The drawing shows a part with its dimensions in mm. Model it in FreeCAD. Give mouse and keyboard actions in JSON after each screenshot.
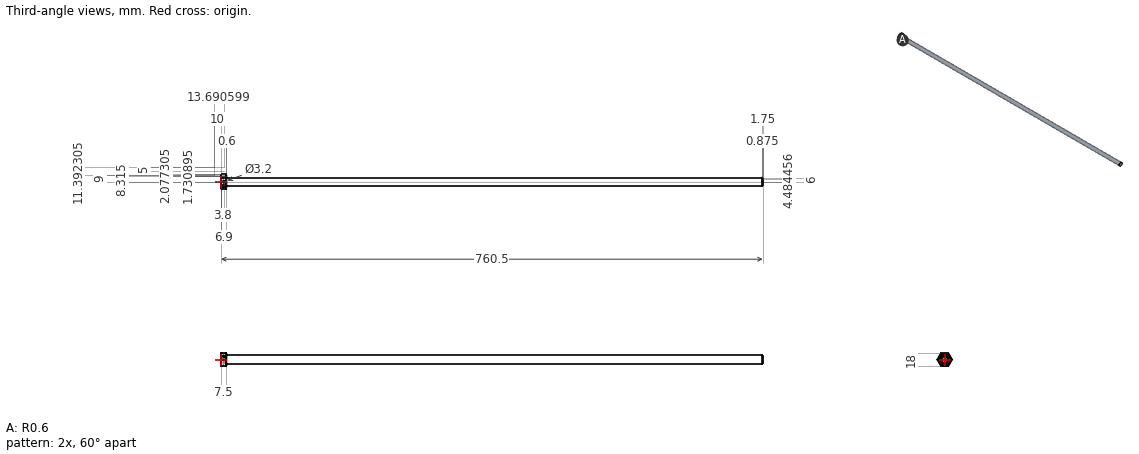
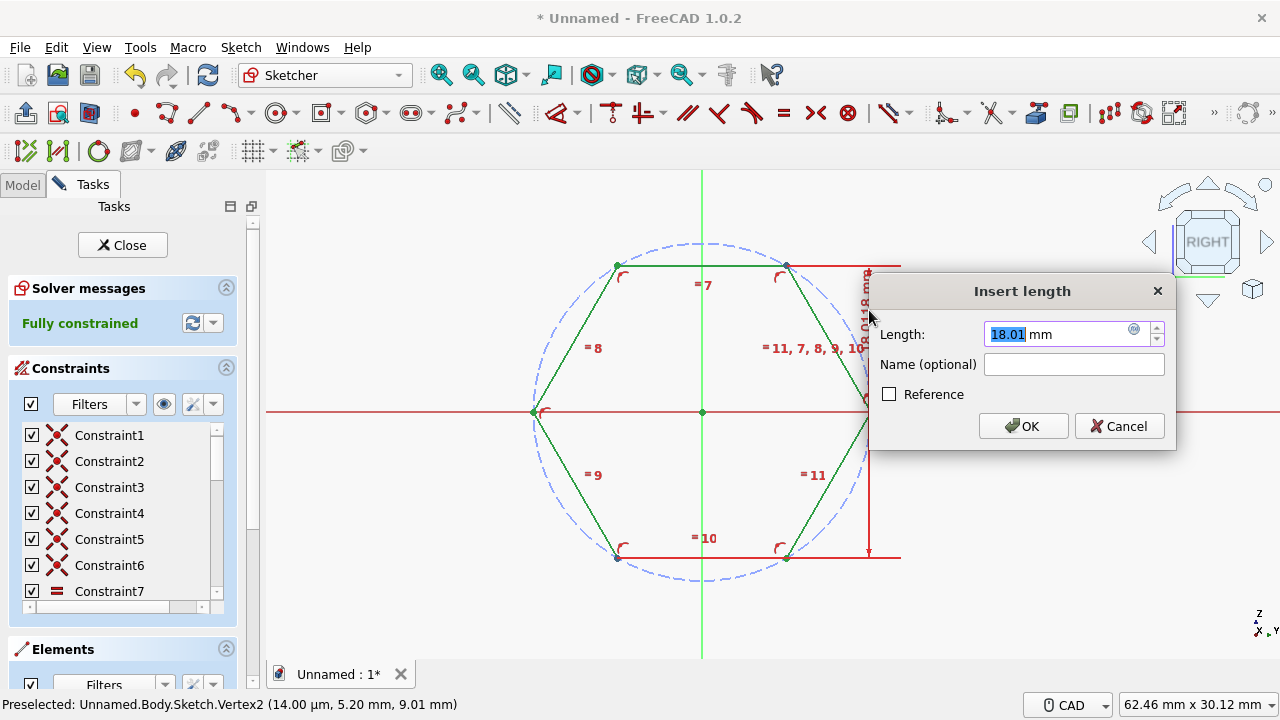
{"action": "type", "text": "18"}
{"action": "key", "text": "Return"}
{"action": "key", "text": "Escape"}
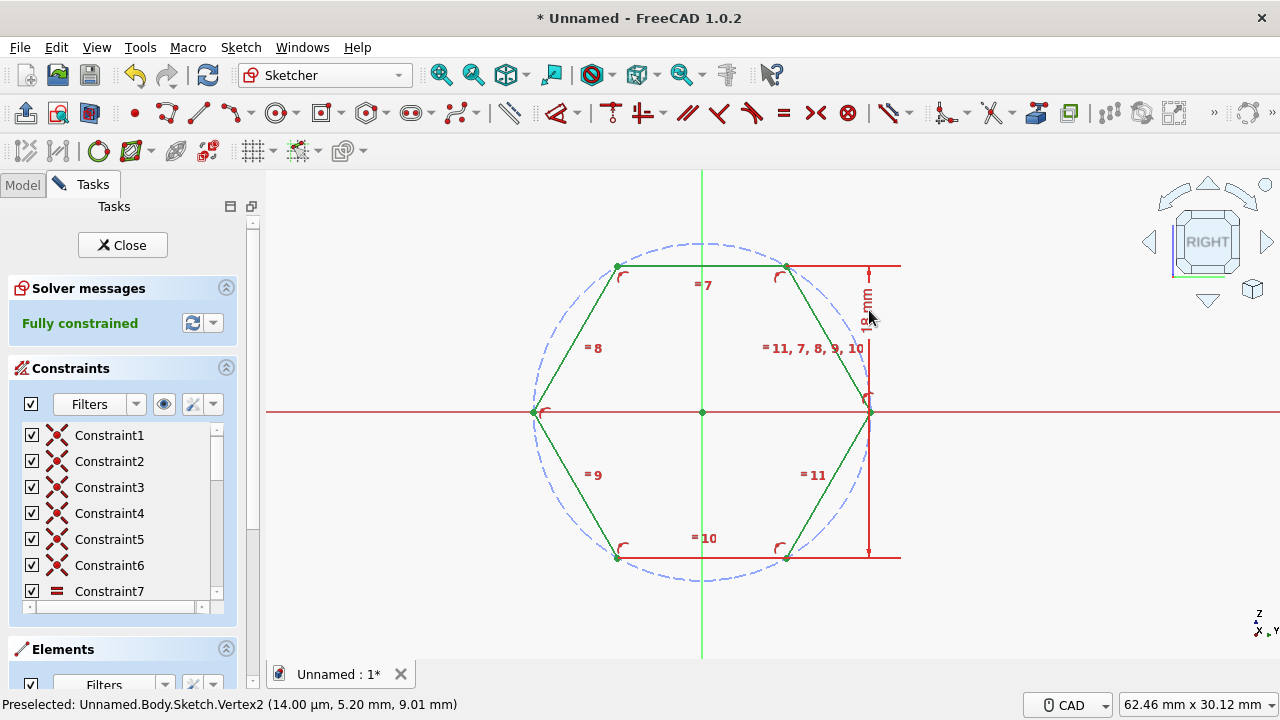
{"action": "left_click", "coordinate": [123, 245]}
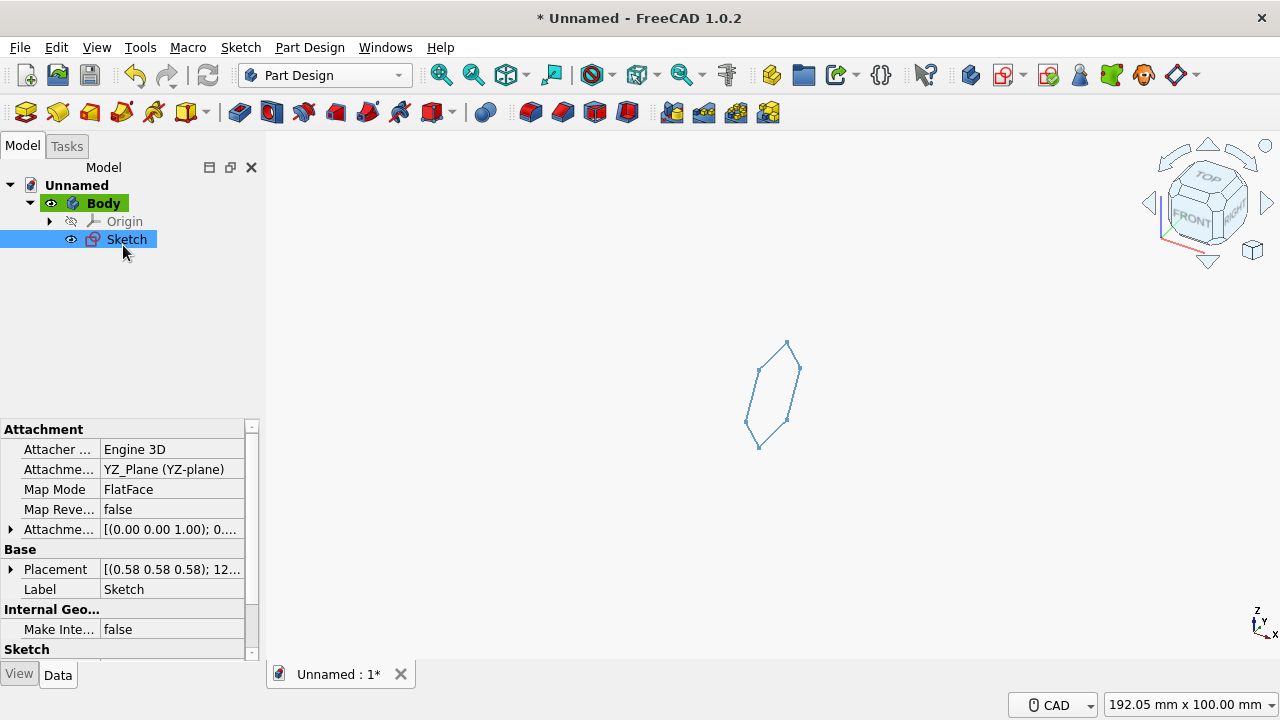
{"action": "left_click", "coordinate": [26, 112]}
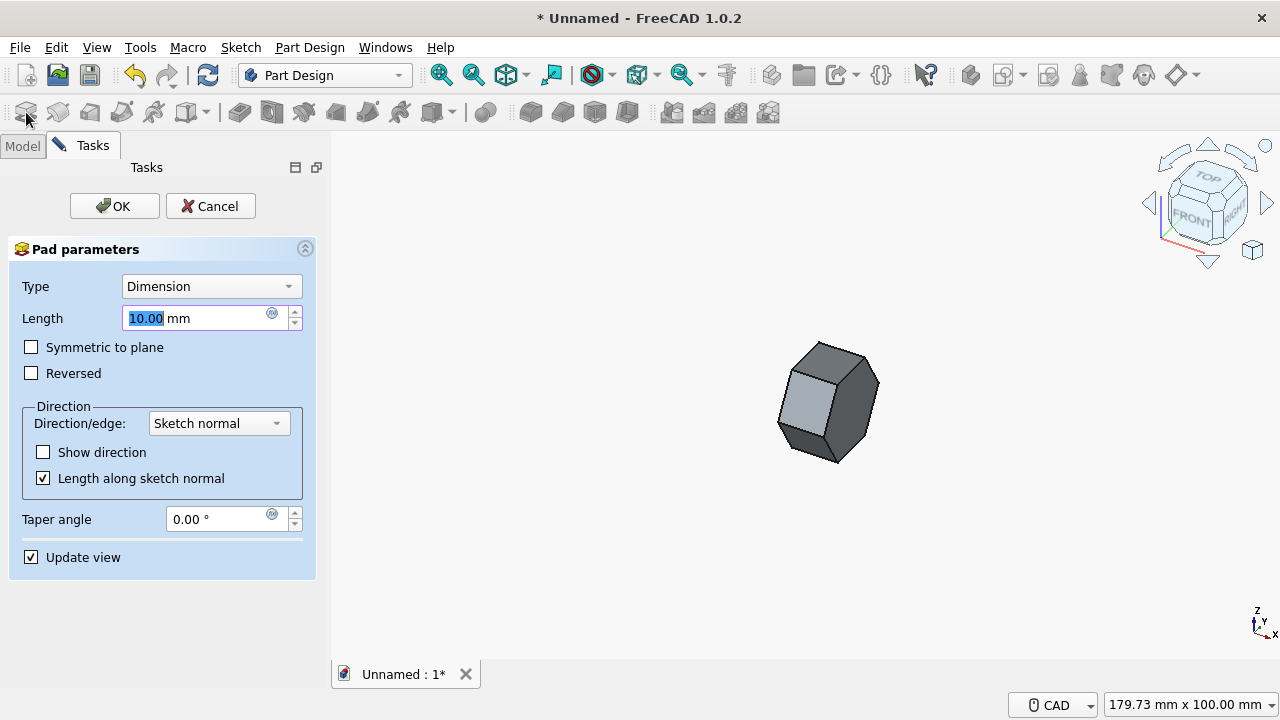
{"action": "type", "text": "7.5"}
{"action": "key", "text": "Tab"}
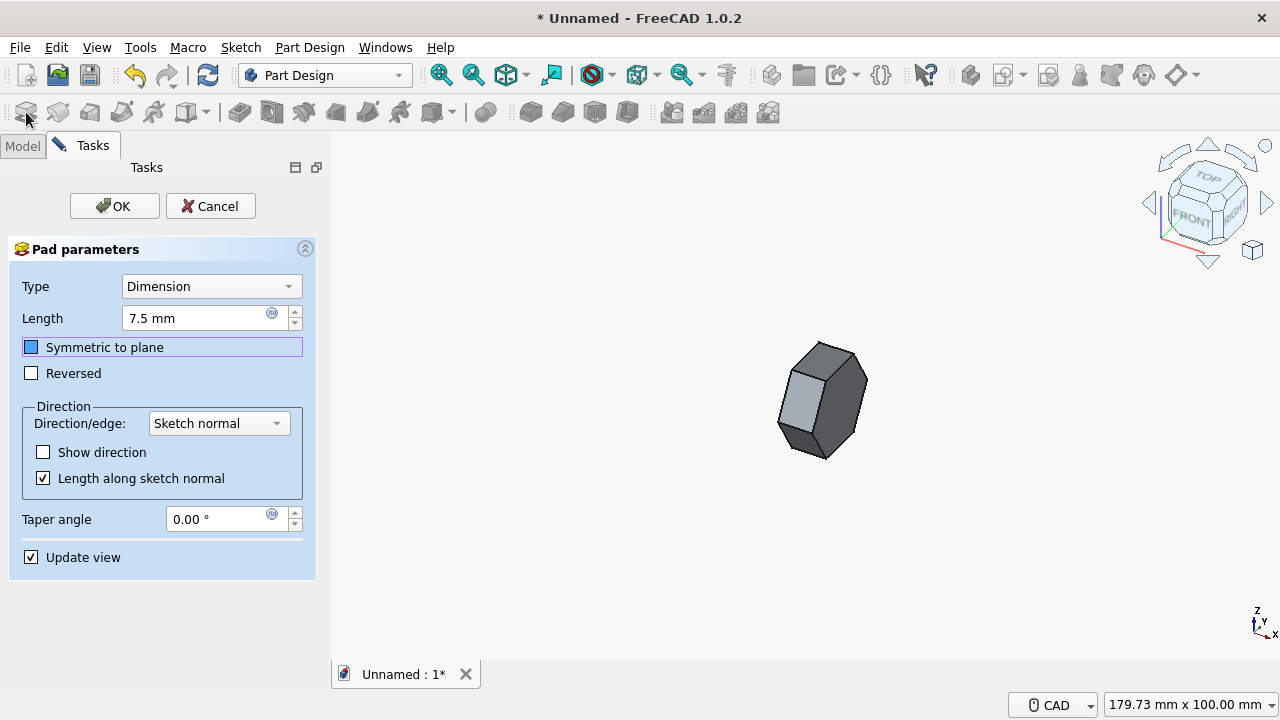
{"action": "left_click", "coordinate": [115, 206]}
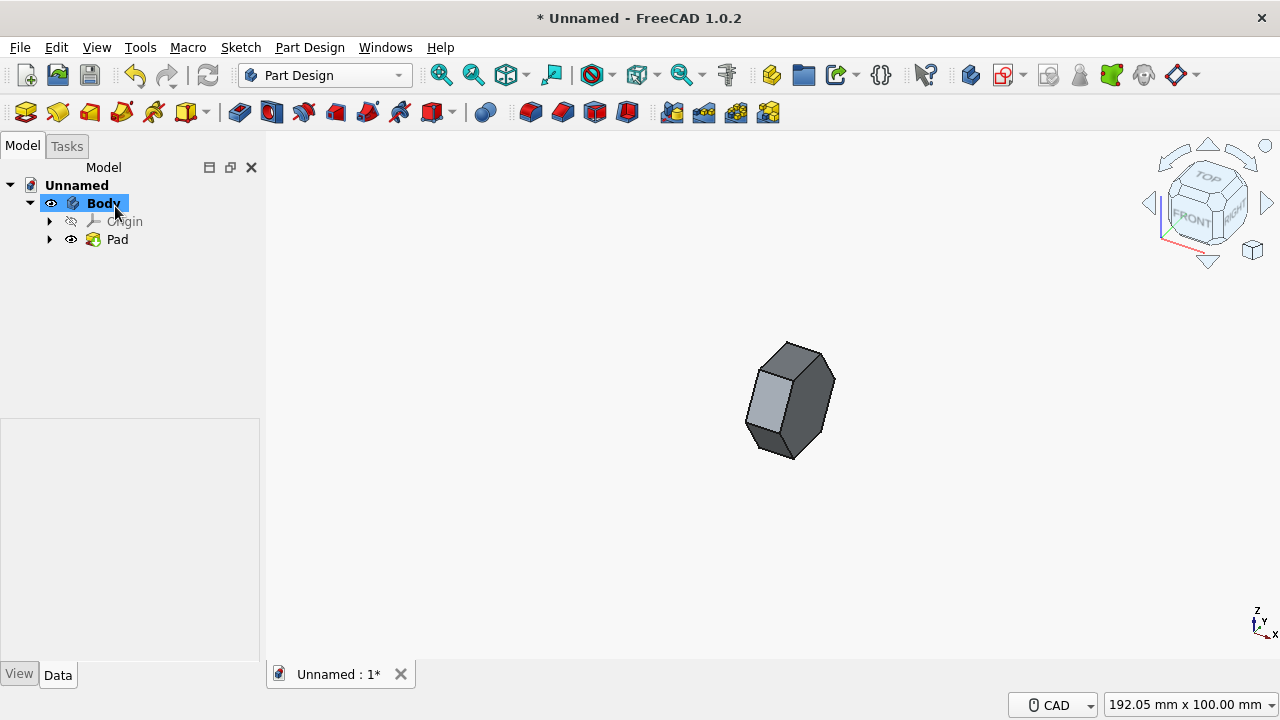
{"action": "left_click", "coordinate": [442, 76]}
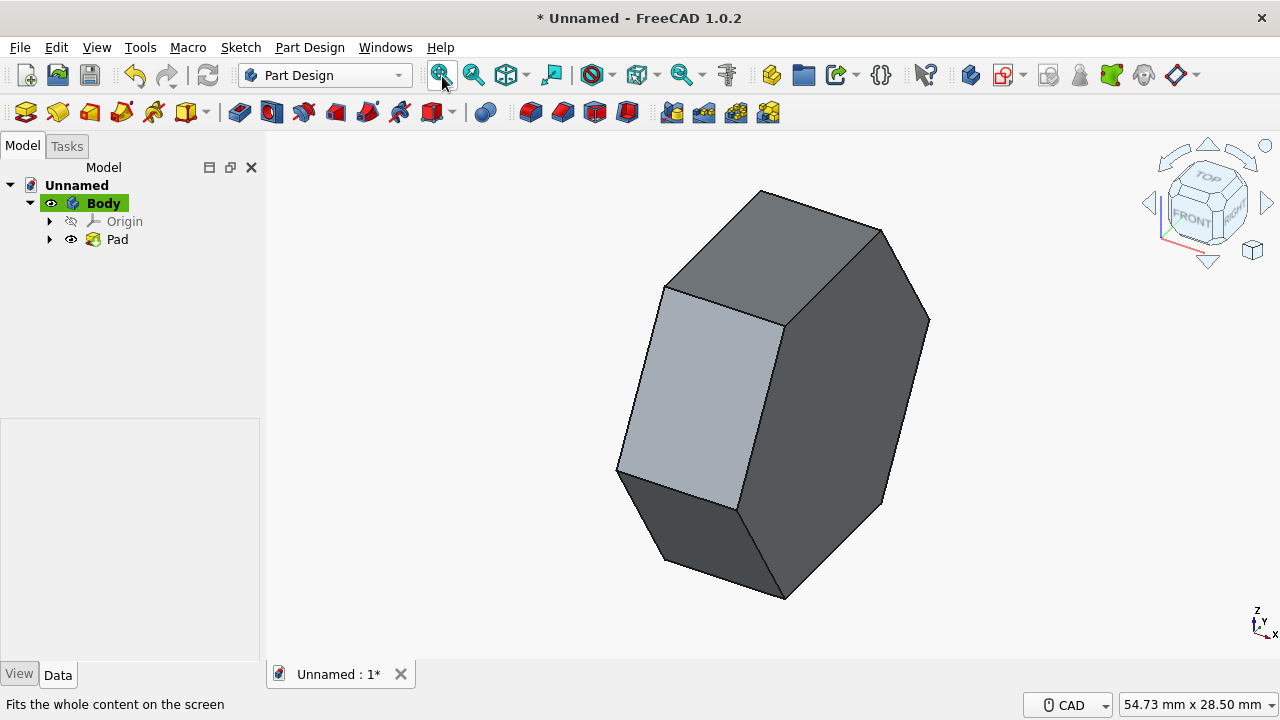
{"action": "left_click", "coordinate": [1004, 76]}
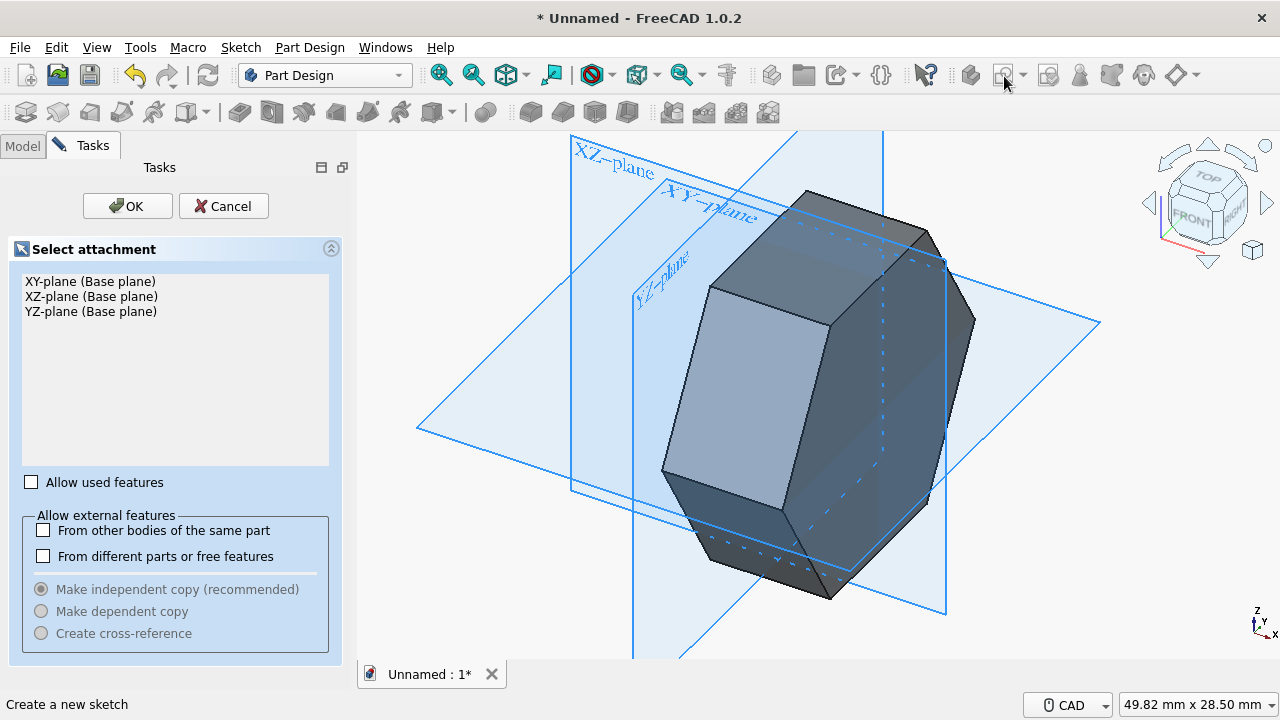
{"action": "left_click", "coordinate": [82, 282]}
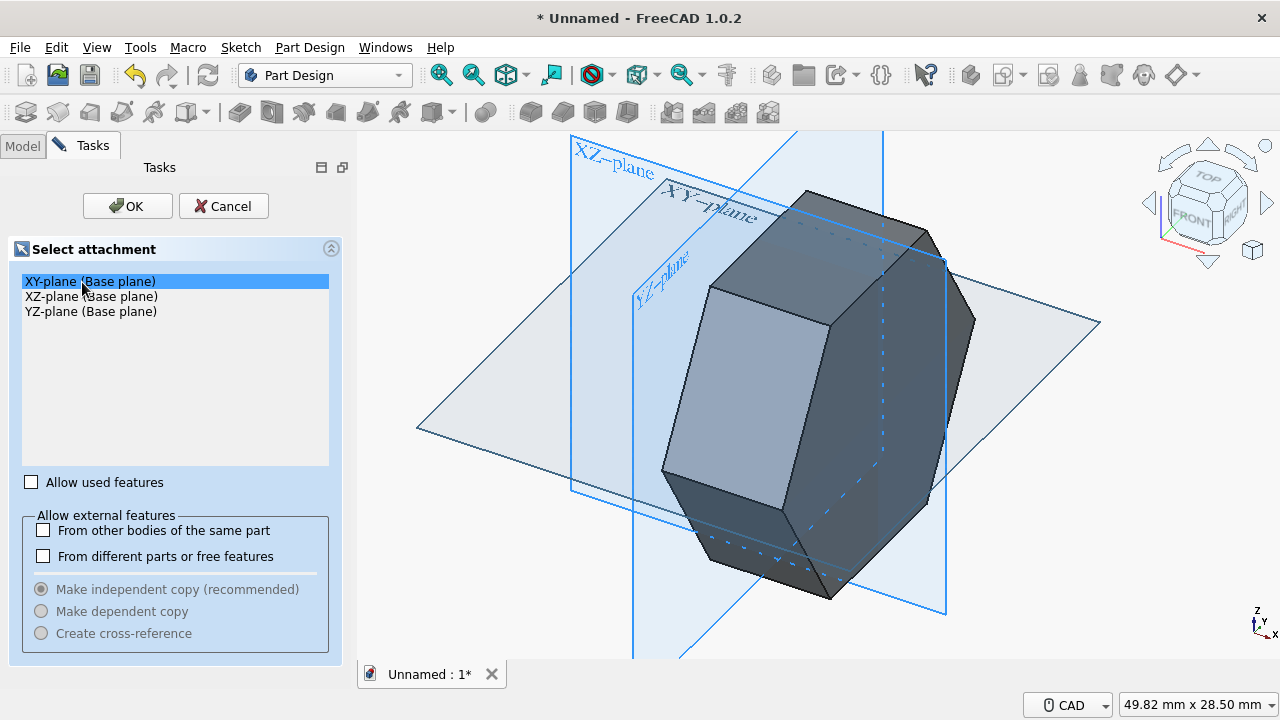
{"action": "left_click", "coordinate": [128, 206]}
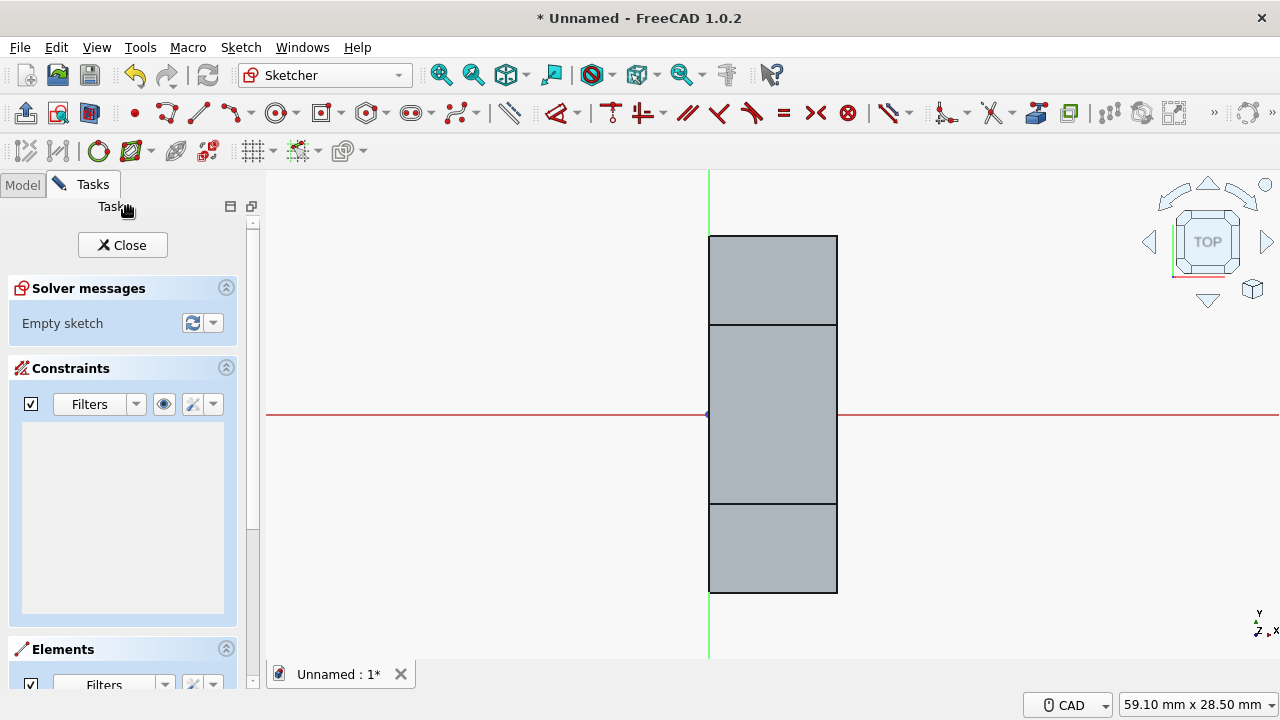
{"action": "key", "text": "q s"}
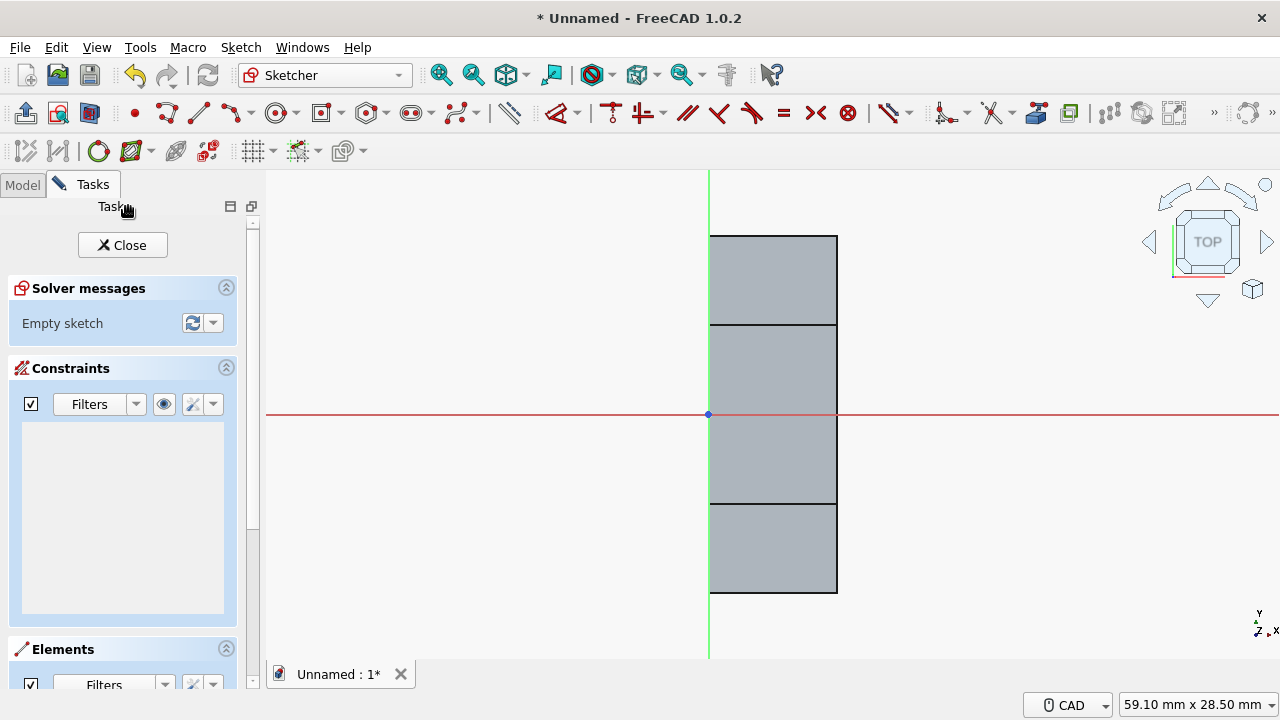
{"action": "scroll", "coordinate": [362, 417], "scroll_direction": "down", "scroll_amount": 15}